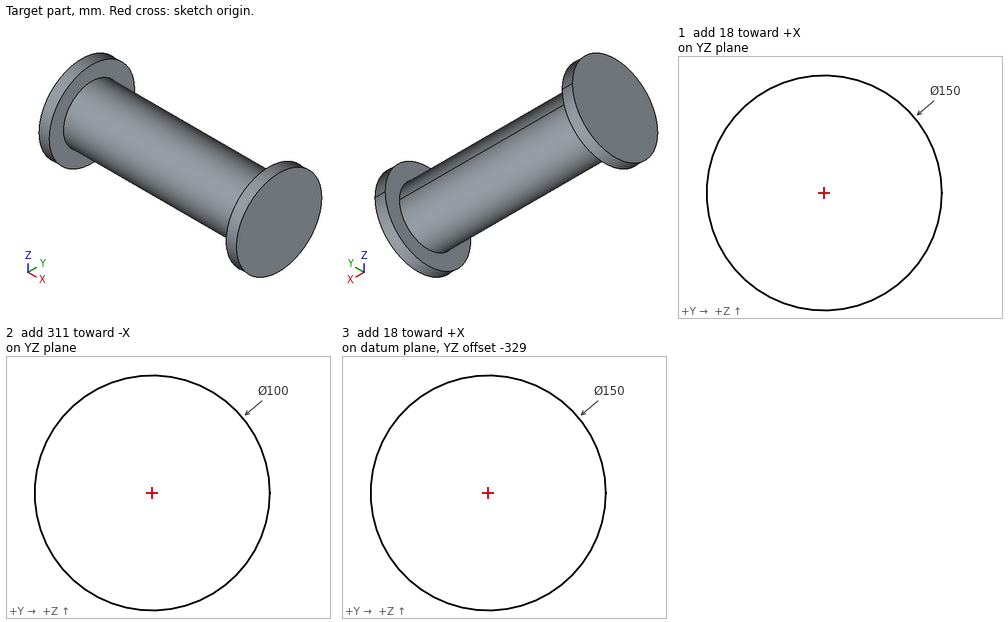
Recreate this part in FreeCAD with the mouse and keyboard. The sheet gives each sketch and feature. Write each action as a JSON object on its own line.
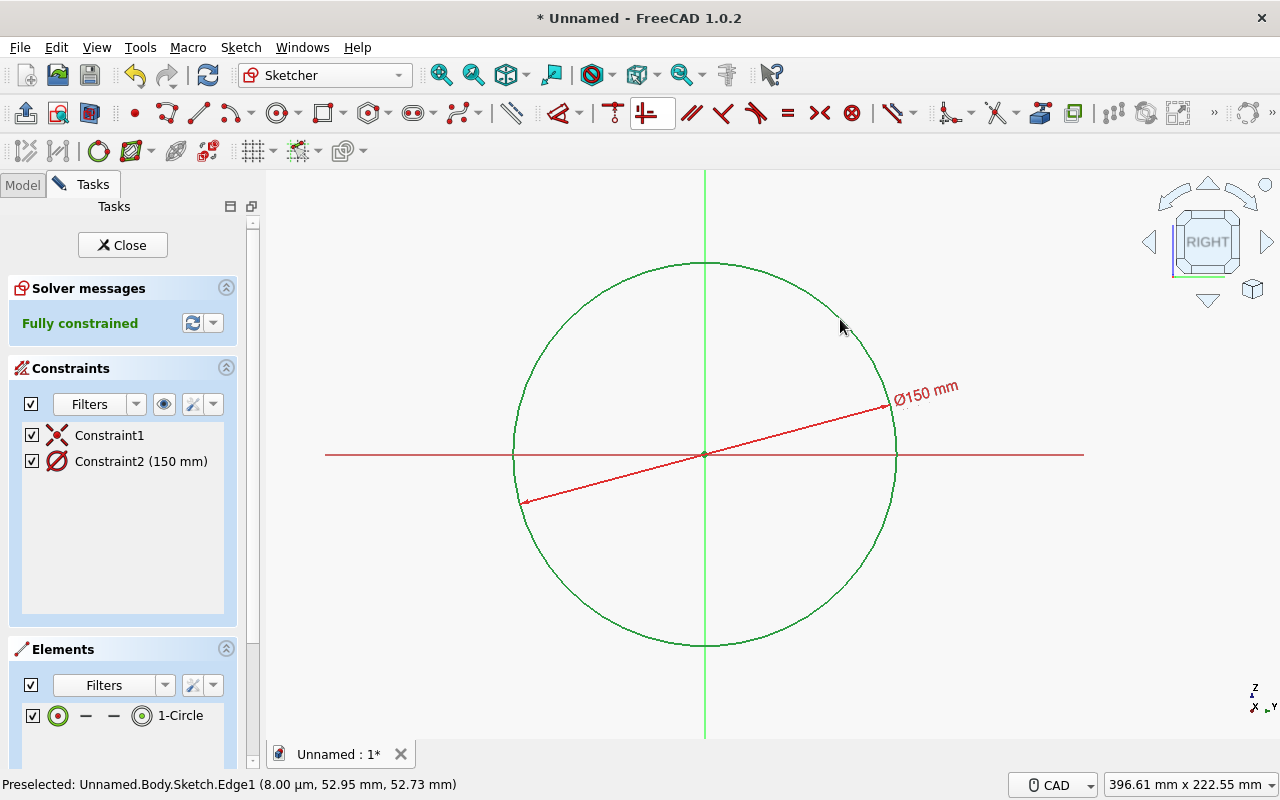
{"action": "left_click", "coordinate": [123, 245]}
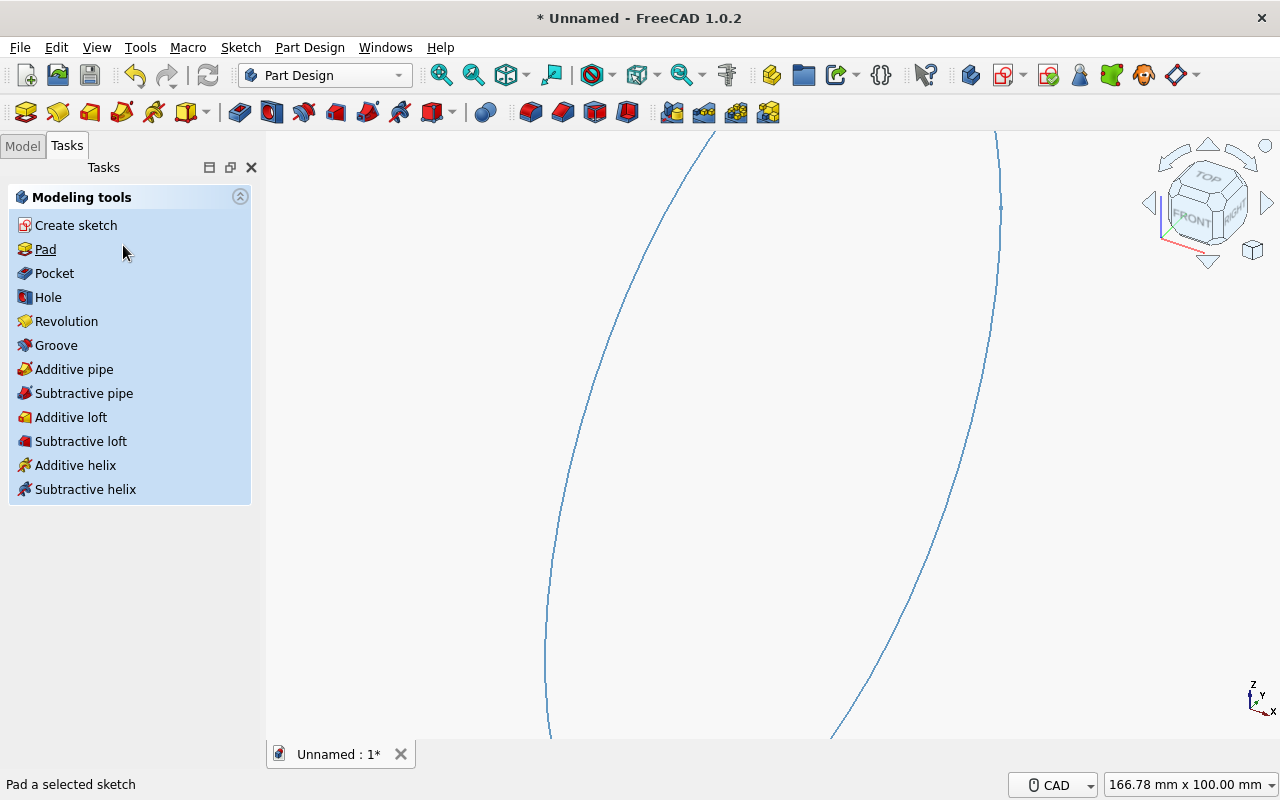
{"action": "left_click", "coordinate": [26, 112]}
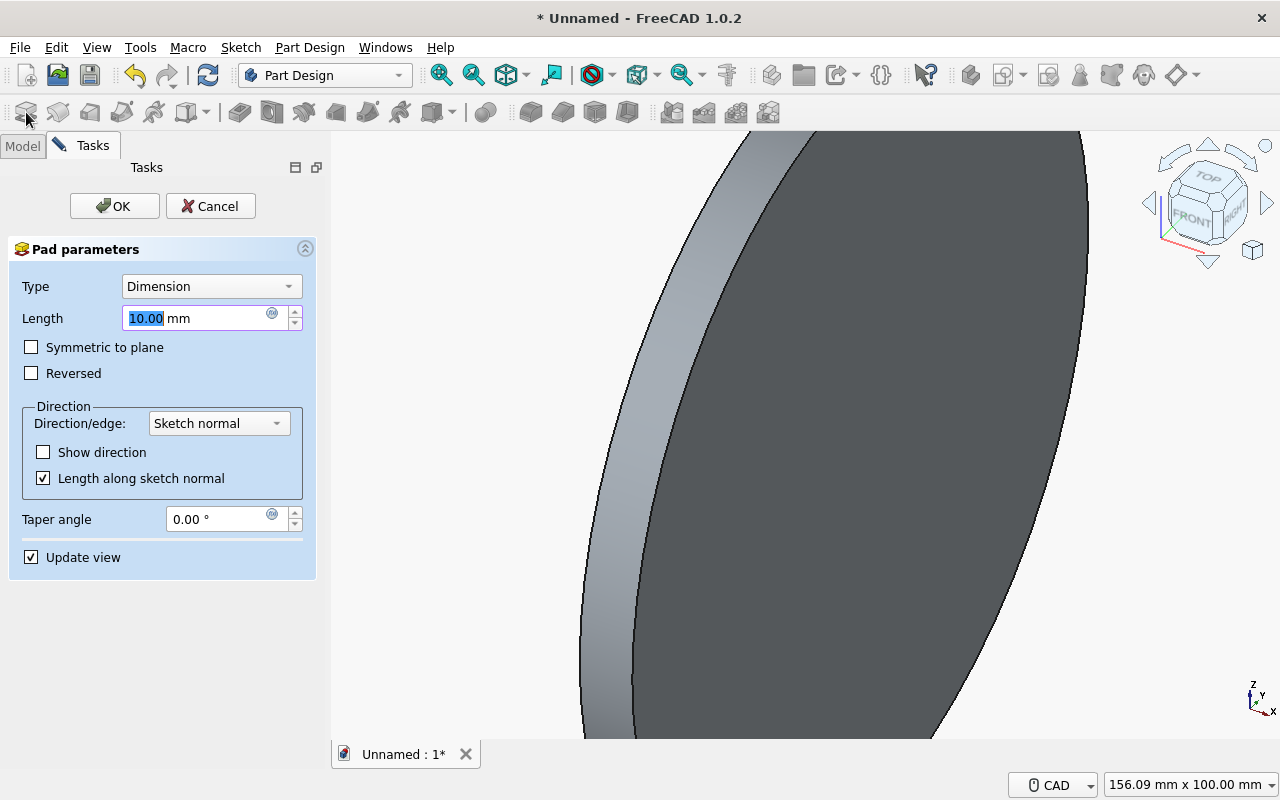
{"action": "type", "text": "18"}
{"action": "key", "text": "Tab"}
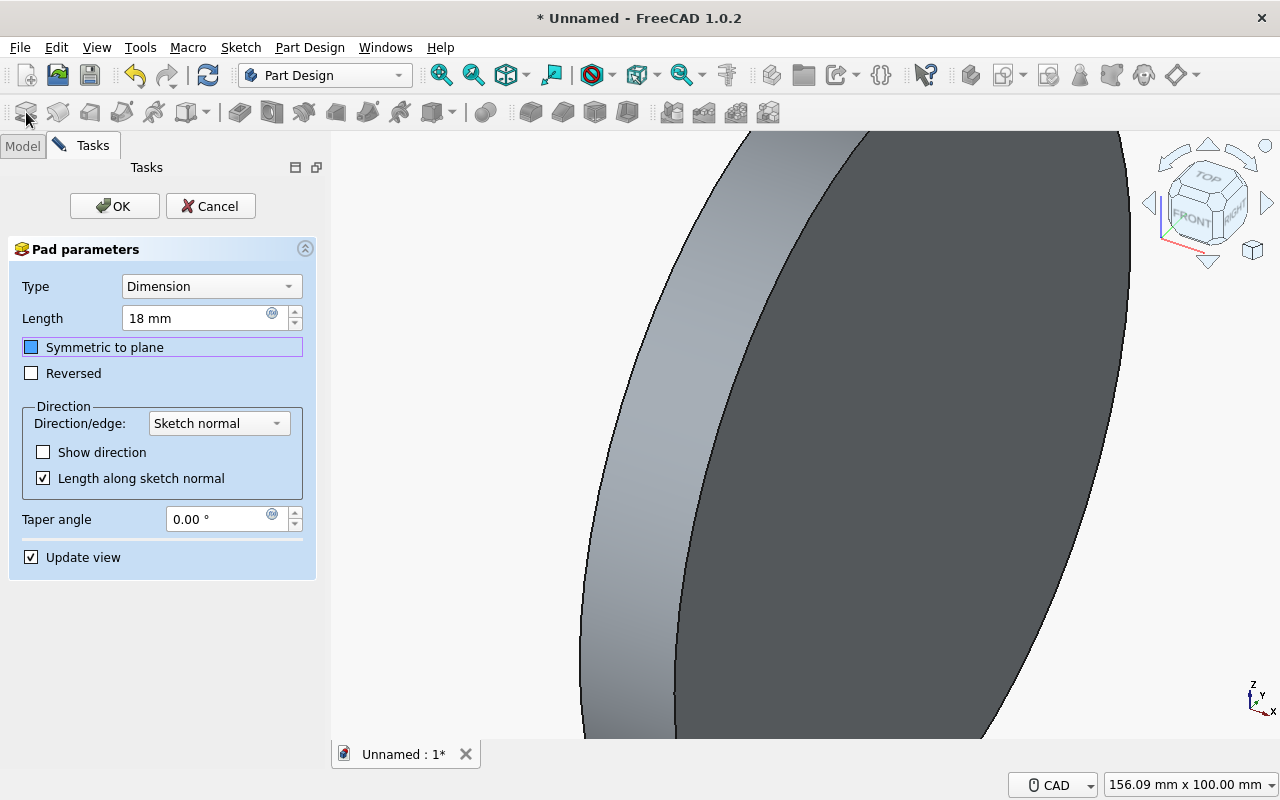
{"action": "left_click", "coordinate": [115, 206]}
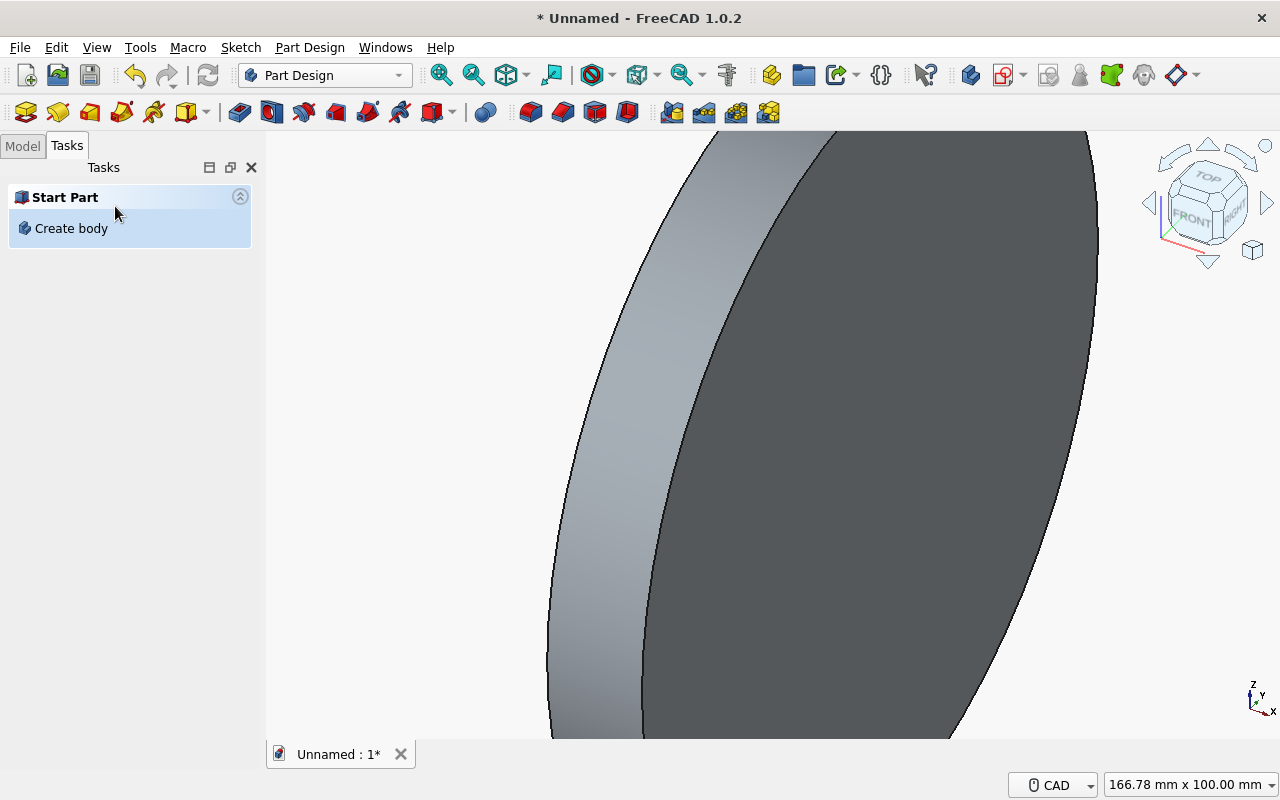
{"action": "left_click", "coordinate": [442, 76]}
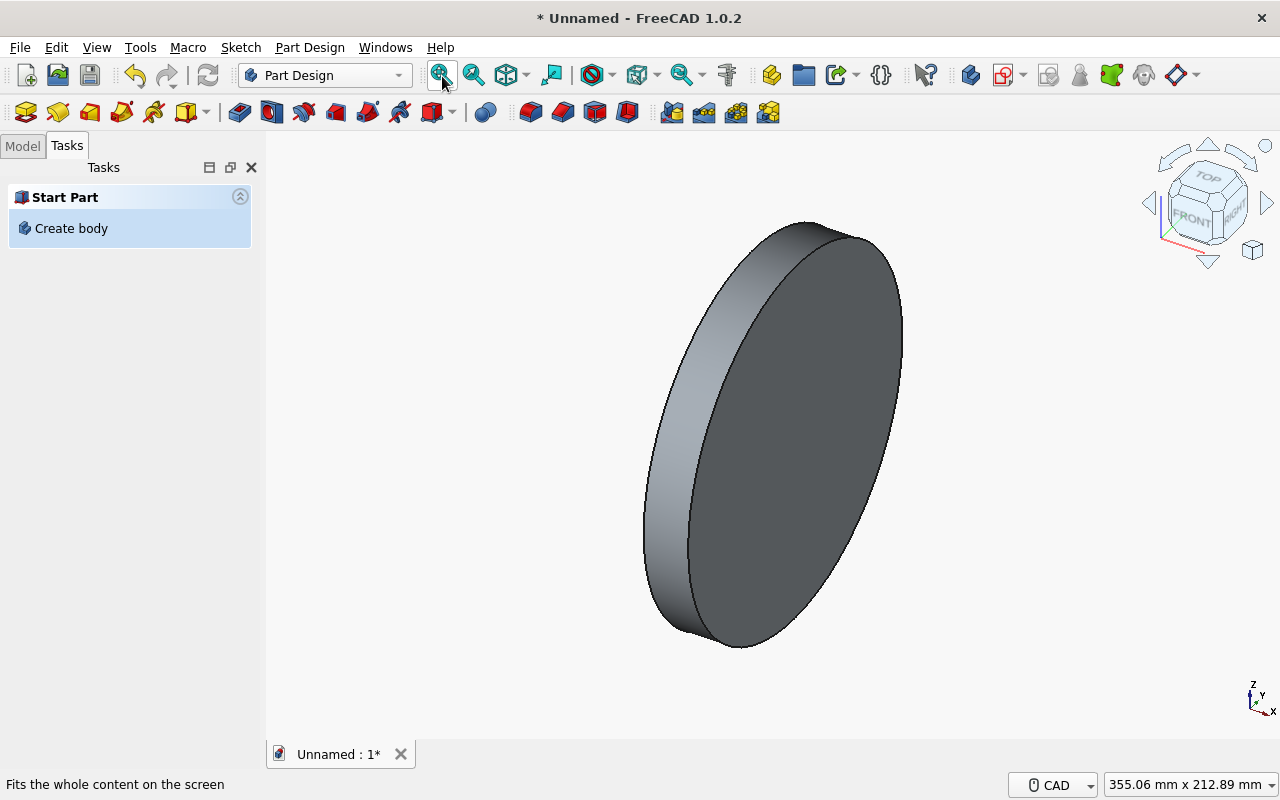
{"action": "left_click", "coordinate": [1004, 76]}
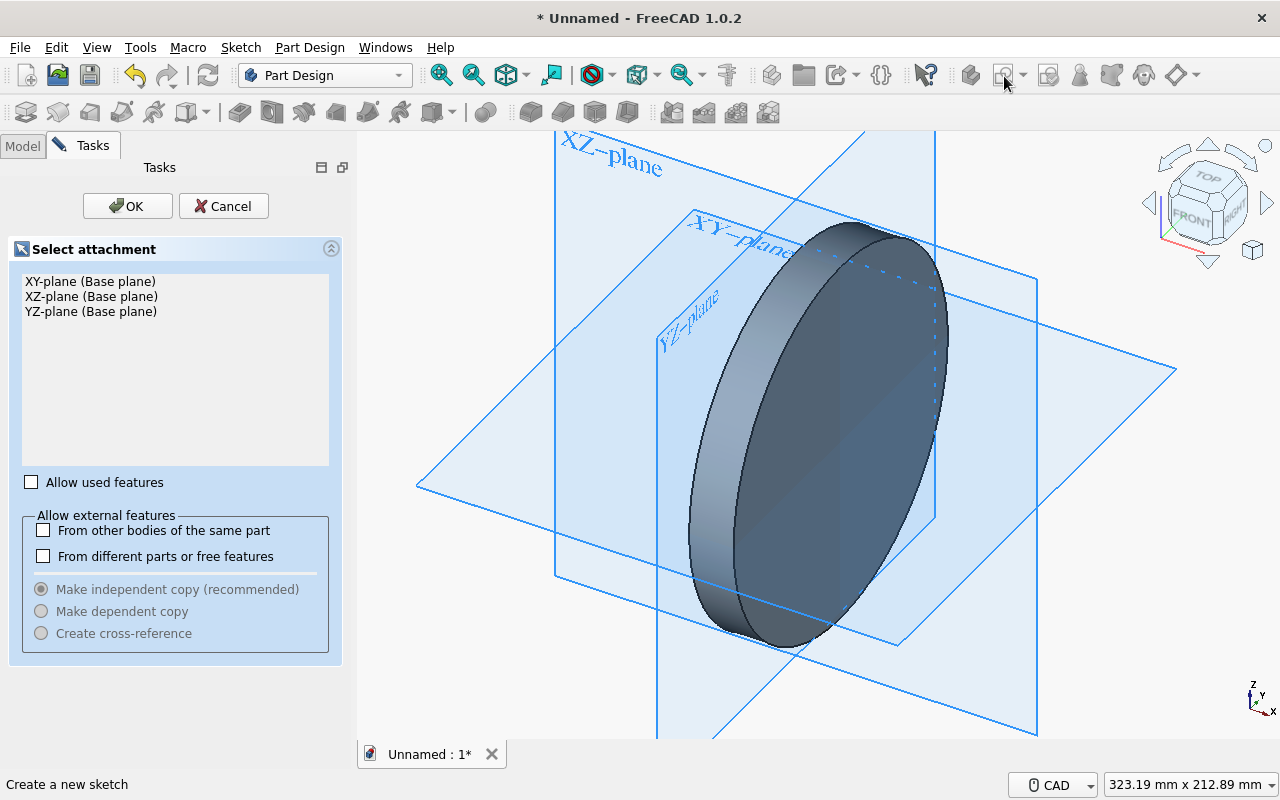
{"action": "left_click", "coordinate": [82, 312]}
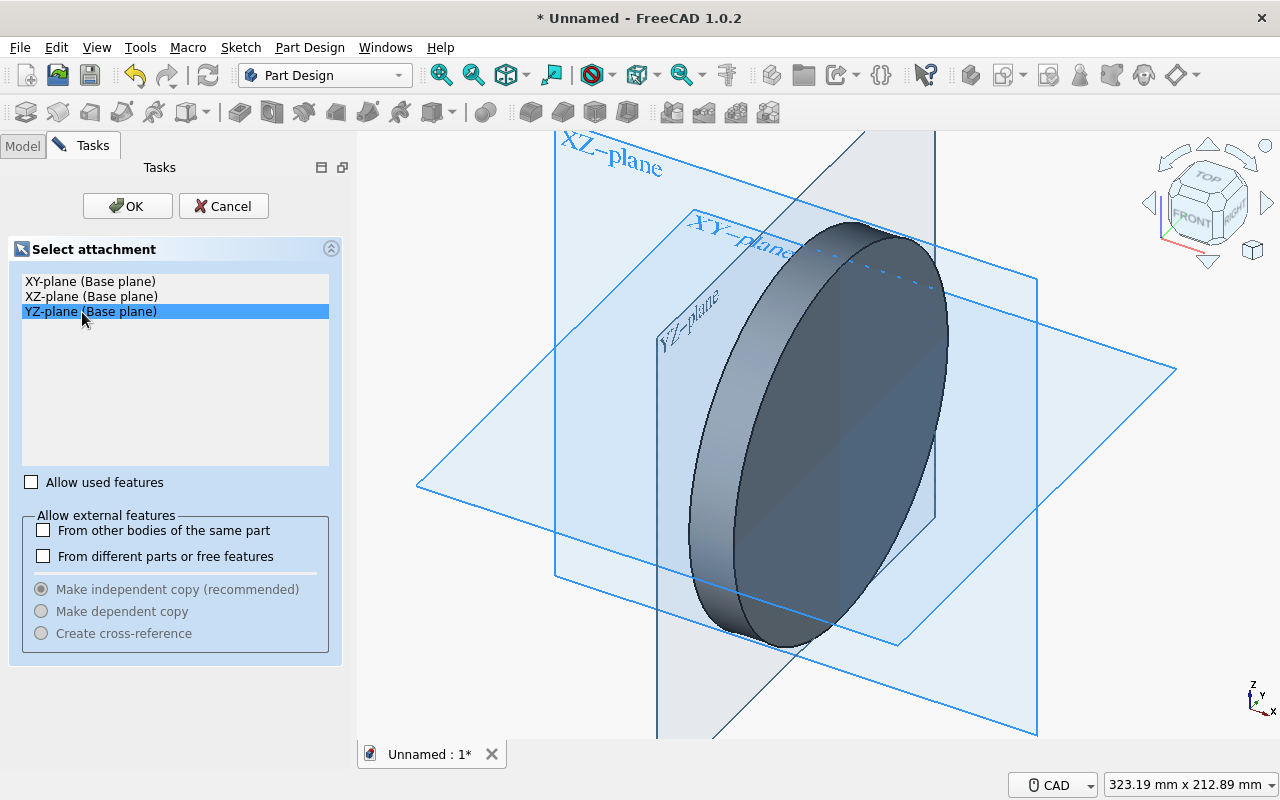
{"action": "left_click", "coordinate": [128, 206]}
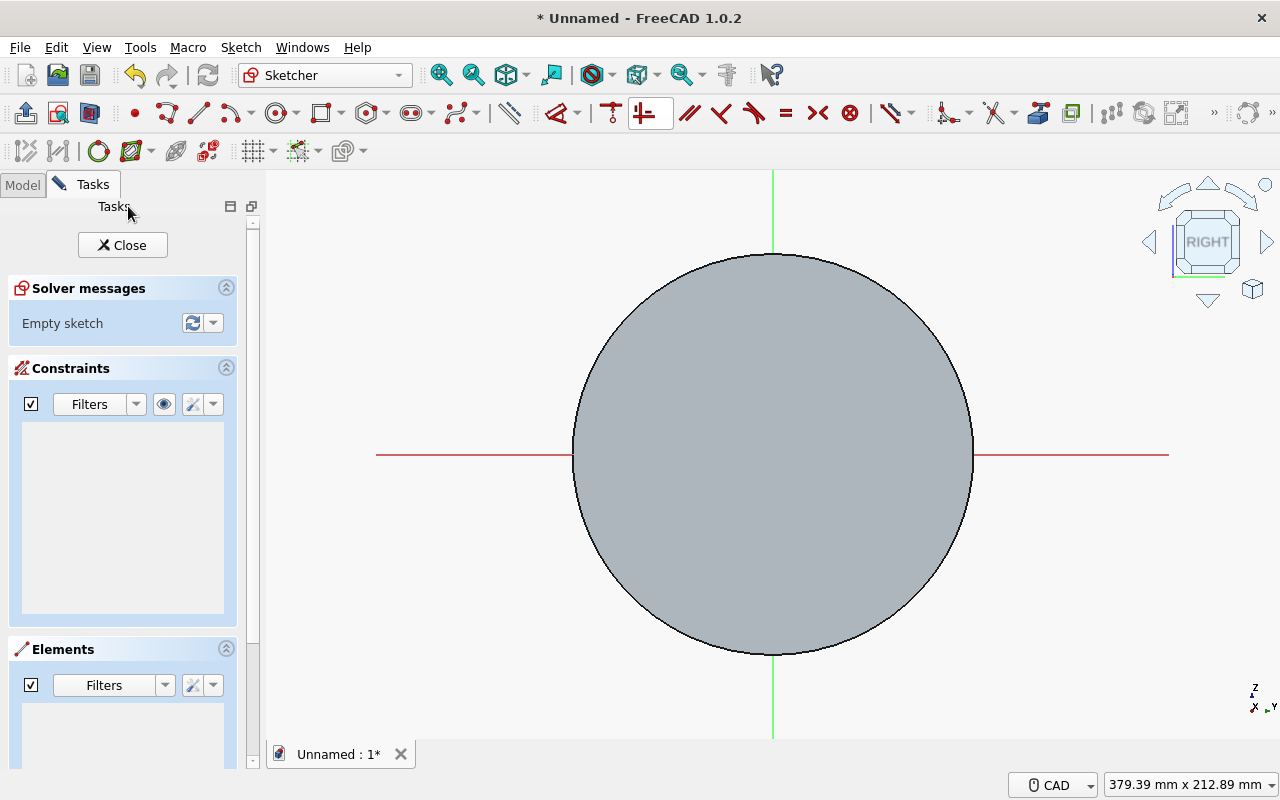
{"action": "left_click", "coordinate": [90, 114]}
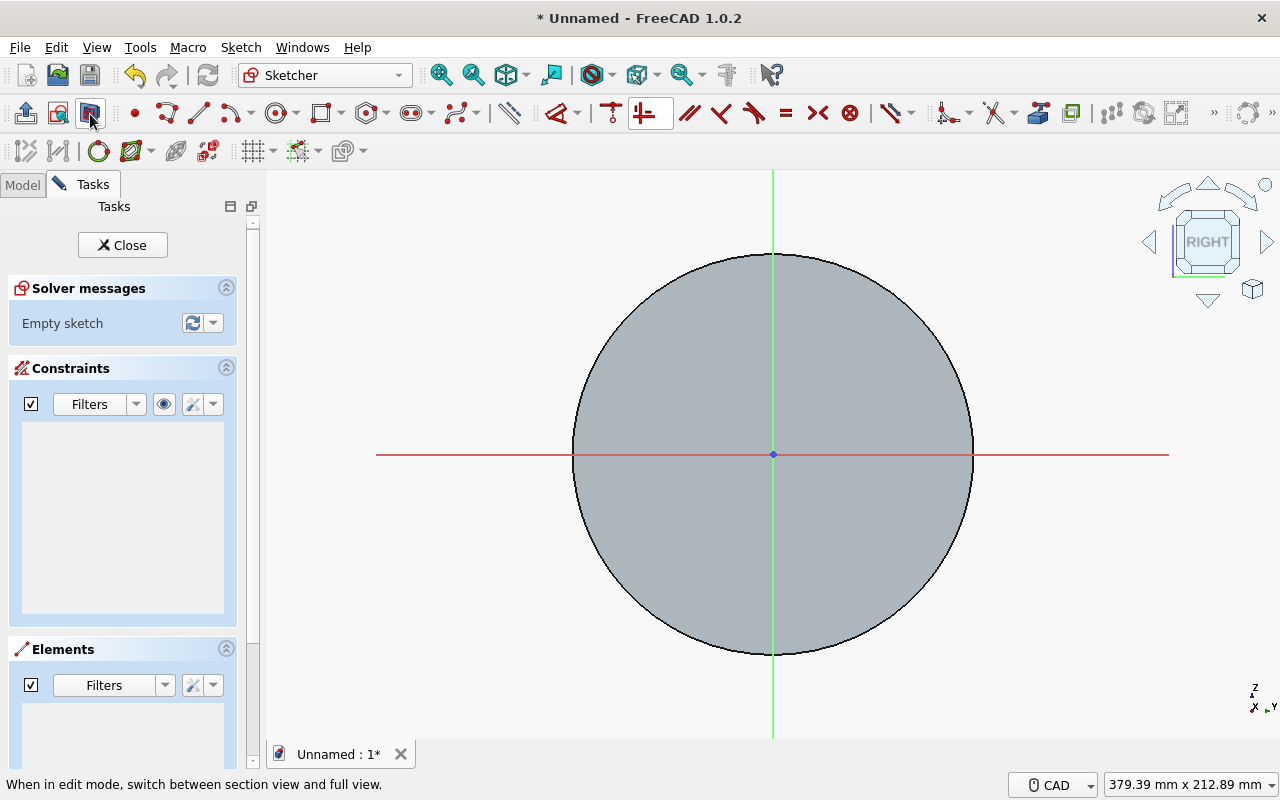
{"action": "scroll", "coordinate": [912, 455], "scroll_direction": "up", "scroll_amount": 2}